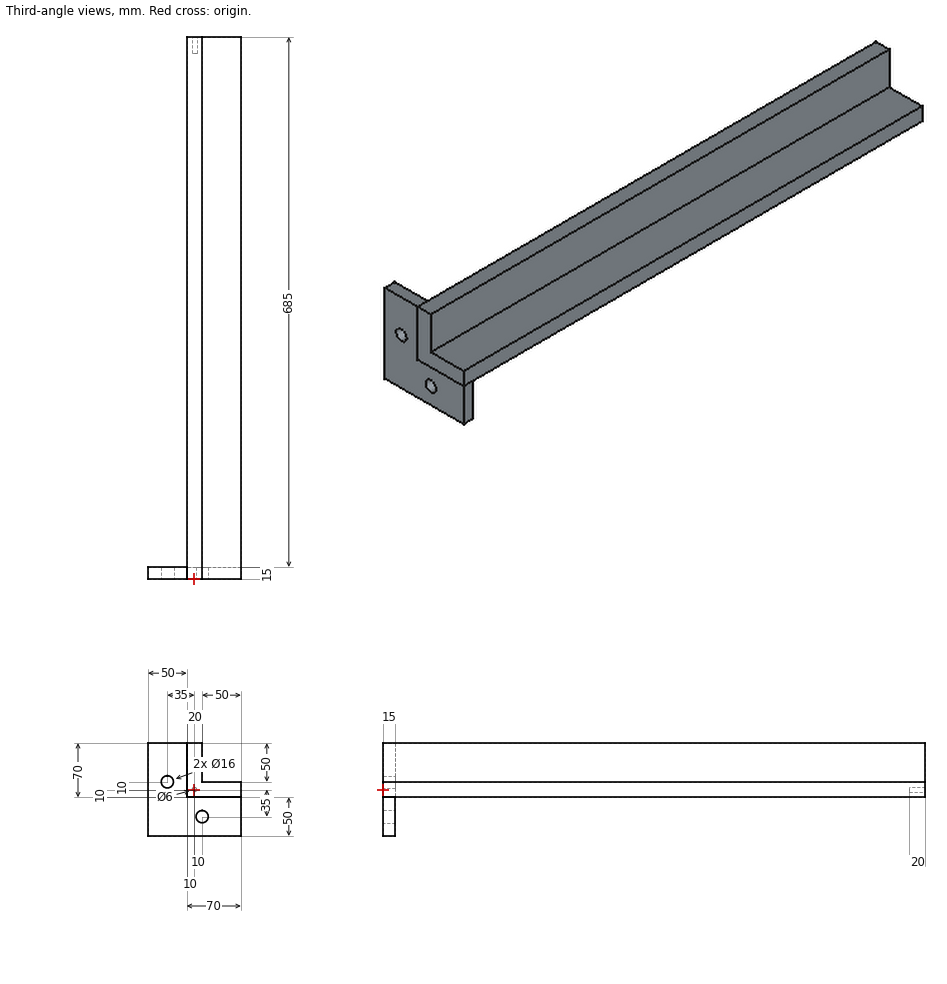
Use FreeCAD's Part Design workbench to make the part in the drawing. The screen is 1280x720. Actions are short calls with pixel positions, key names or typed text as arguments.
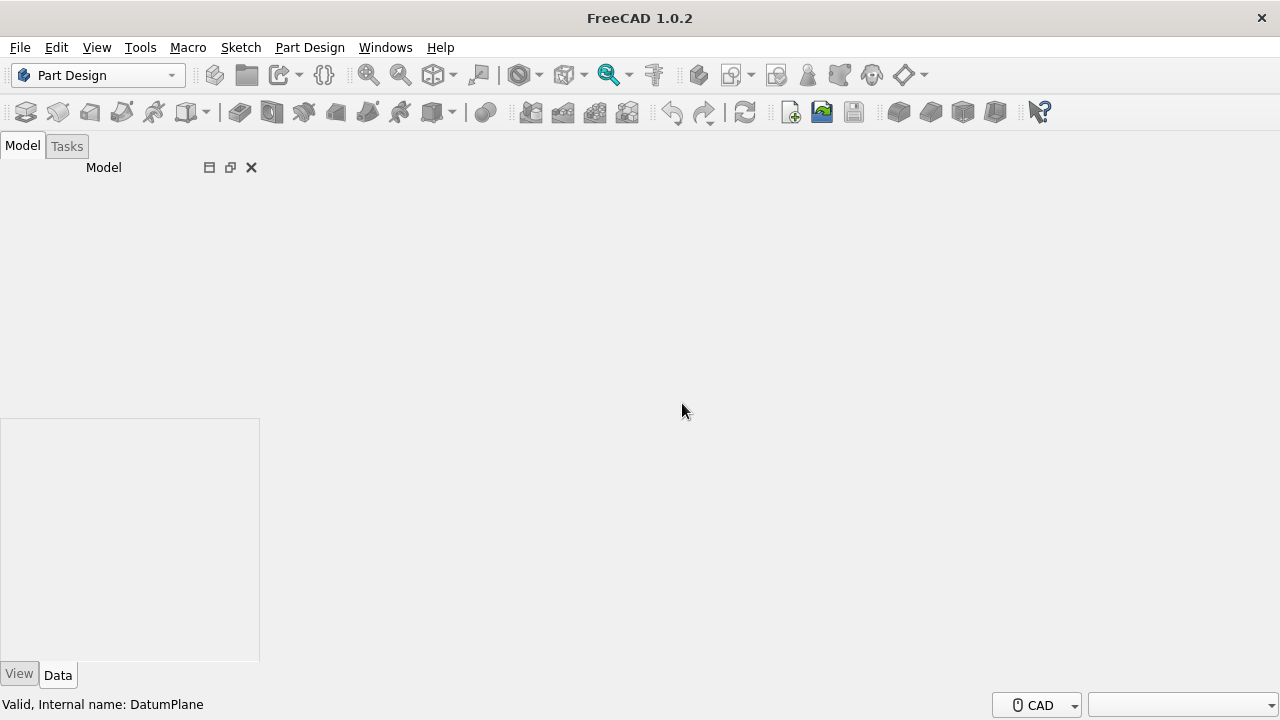
click(790, 112)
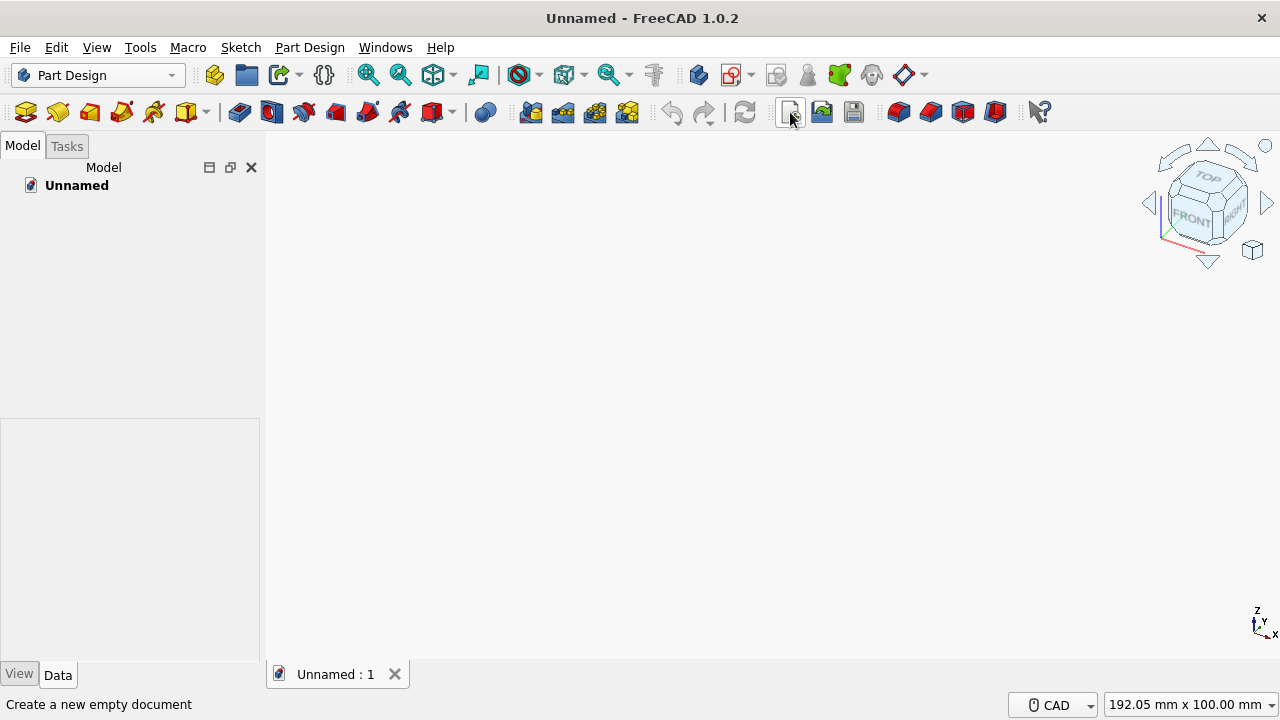
click(732, 76)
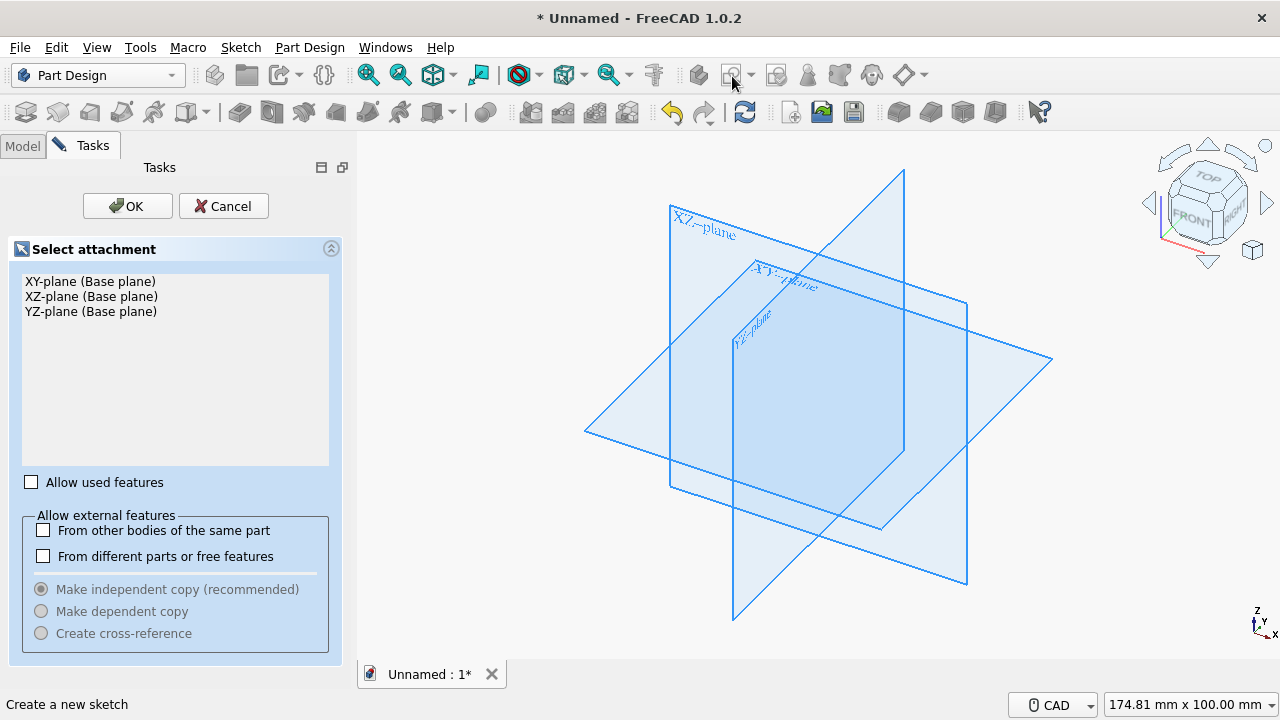
click(82, 296)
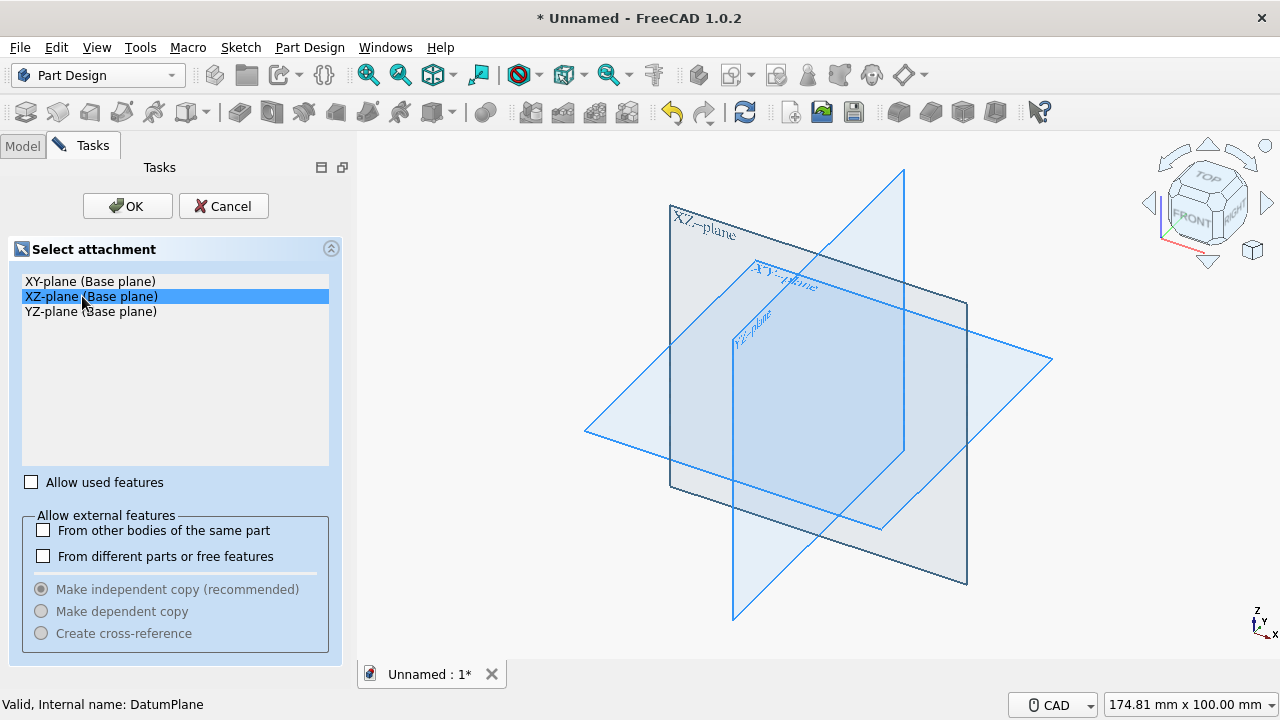
click(128, 206)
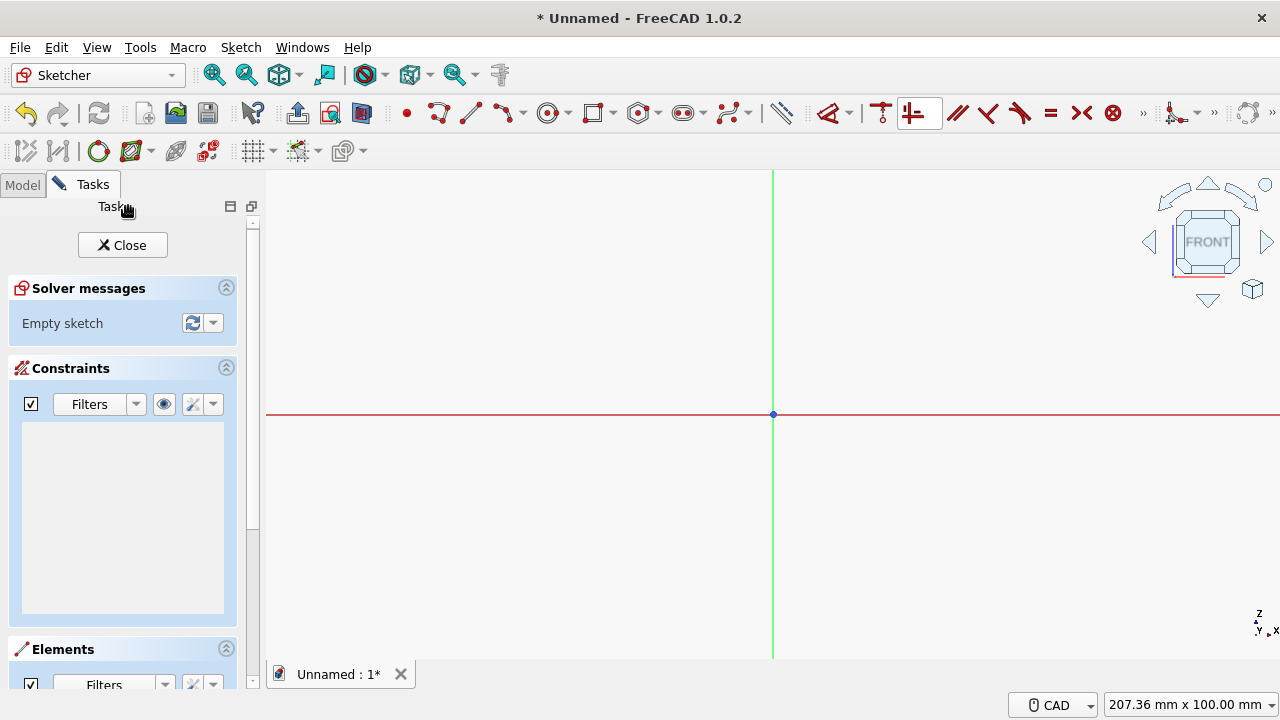
scroll(621, 414, down, 3)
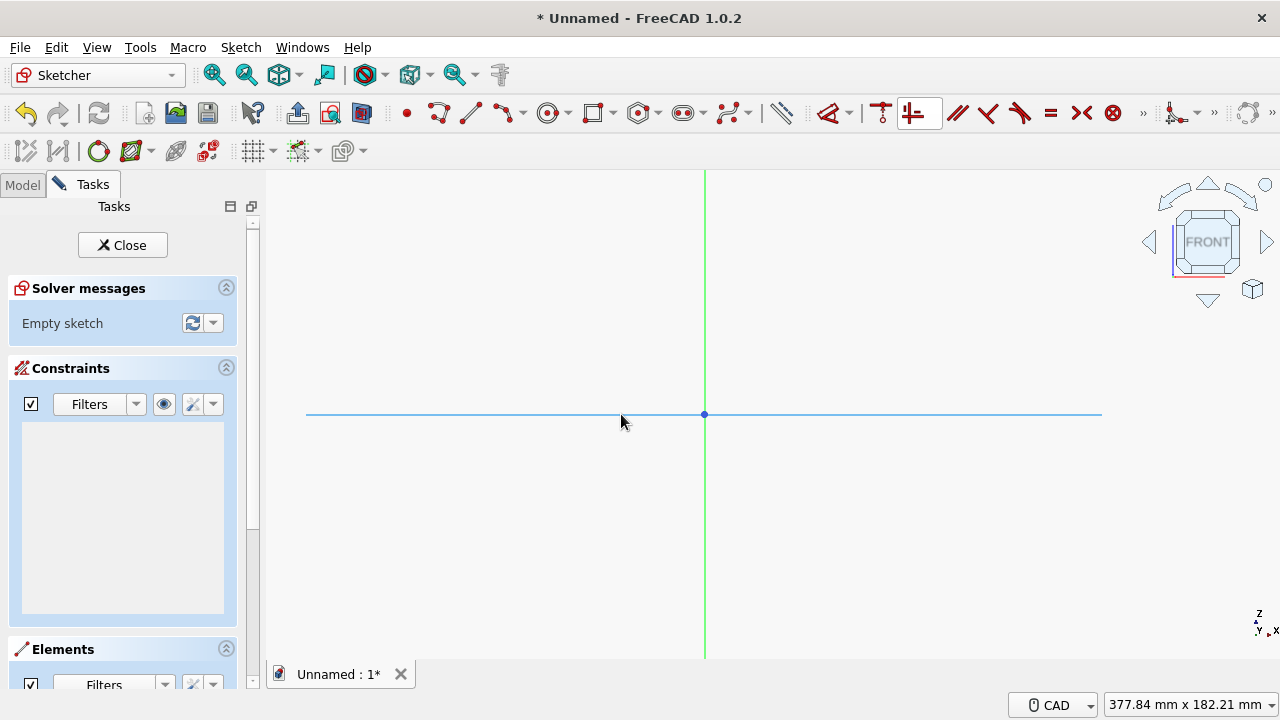
click(440, 114)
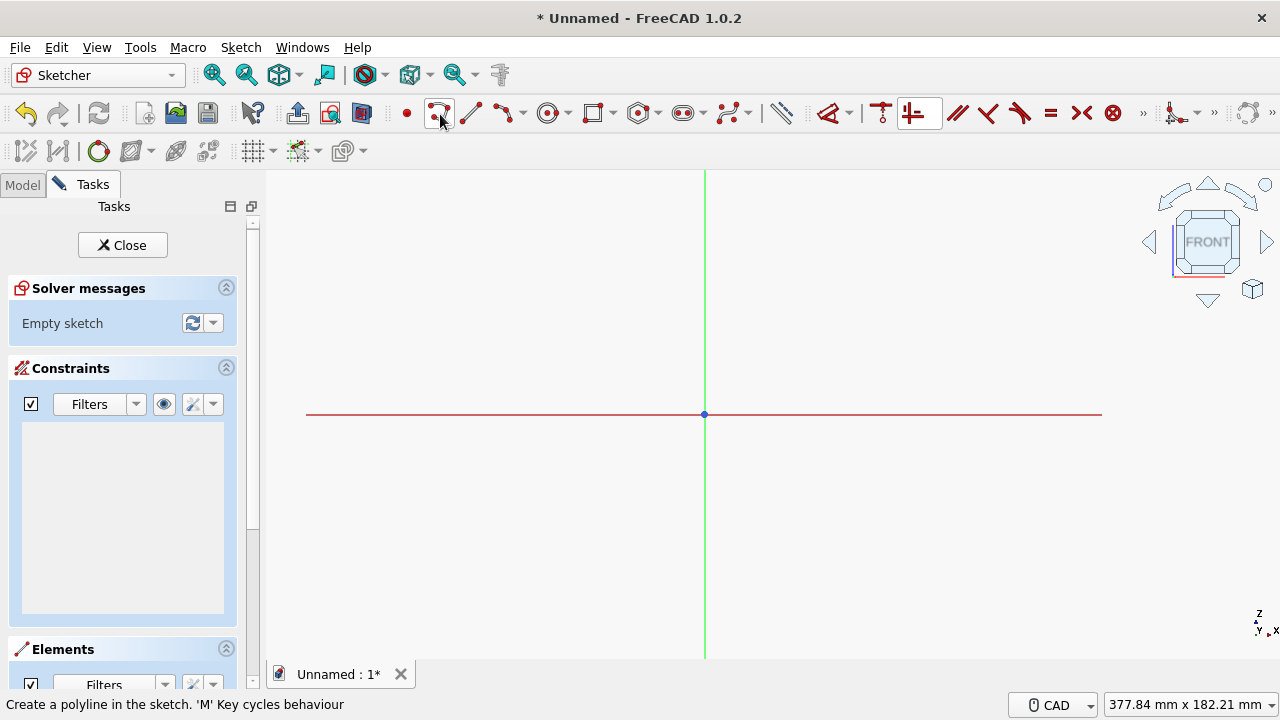
click(678, 441)
click(866, 441)
click(866, 576)
click(544, 576)
click(544, 253)
click(678, 253)
click(678, 442)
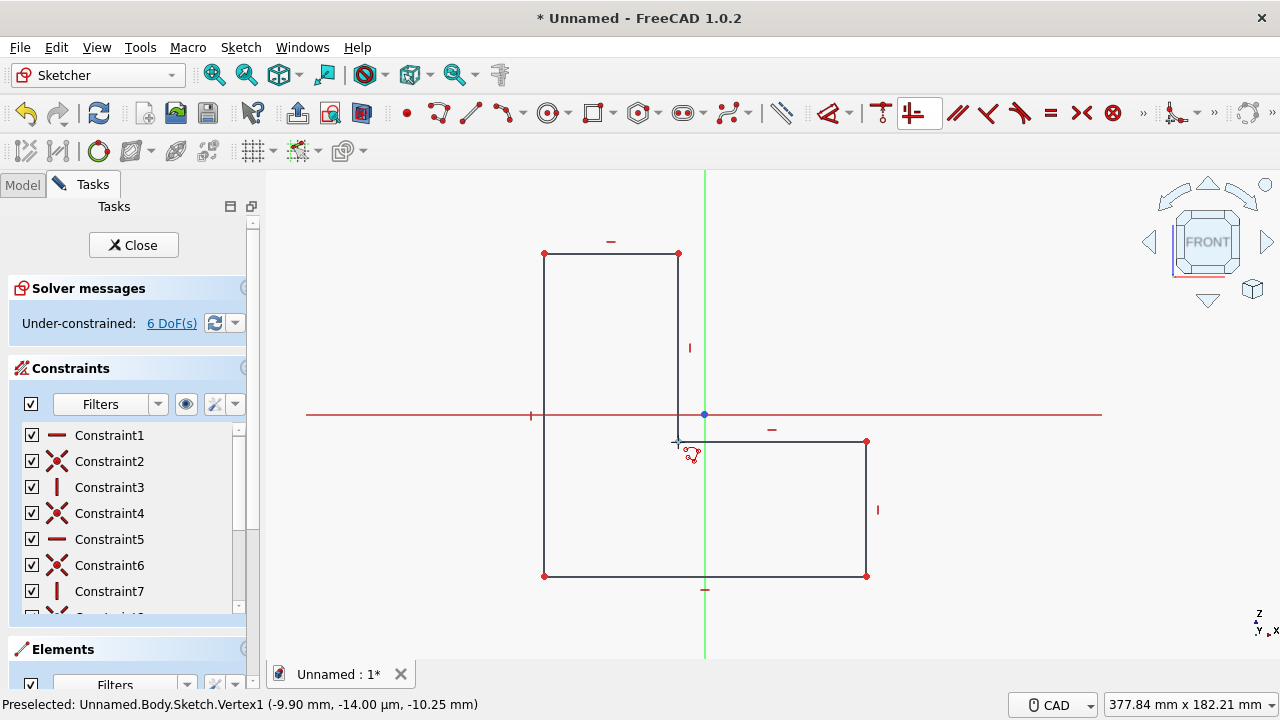
click(548, 114)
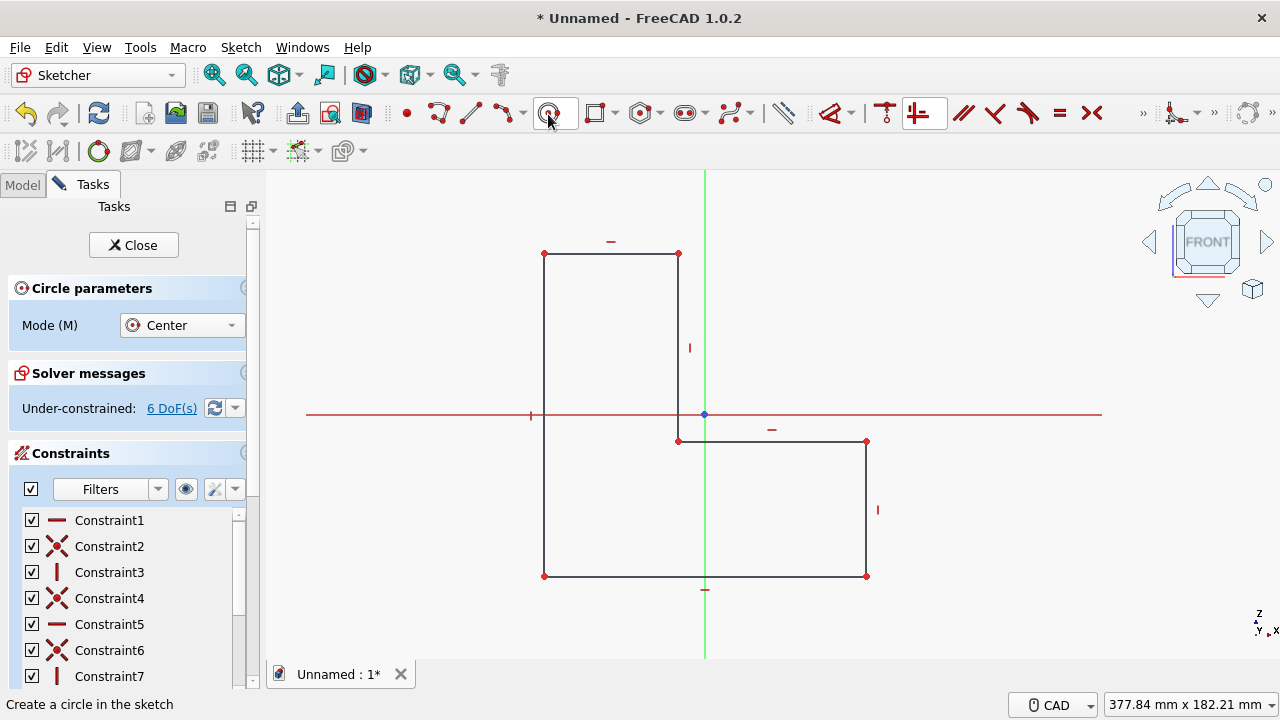
click(611, 388)
move(626, 372)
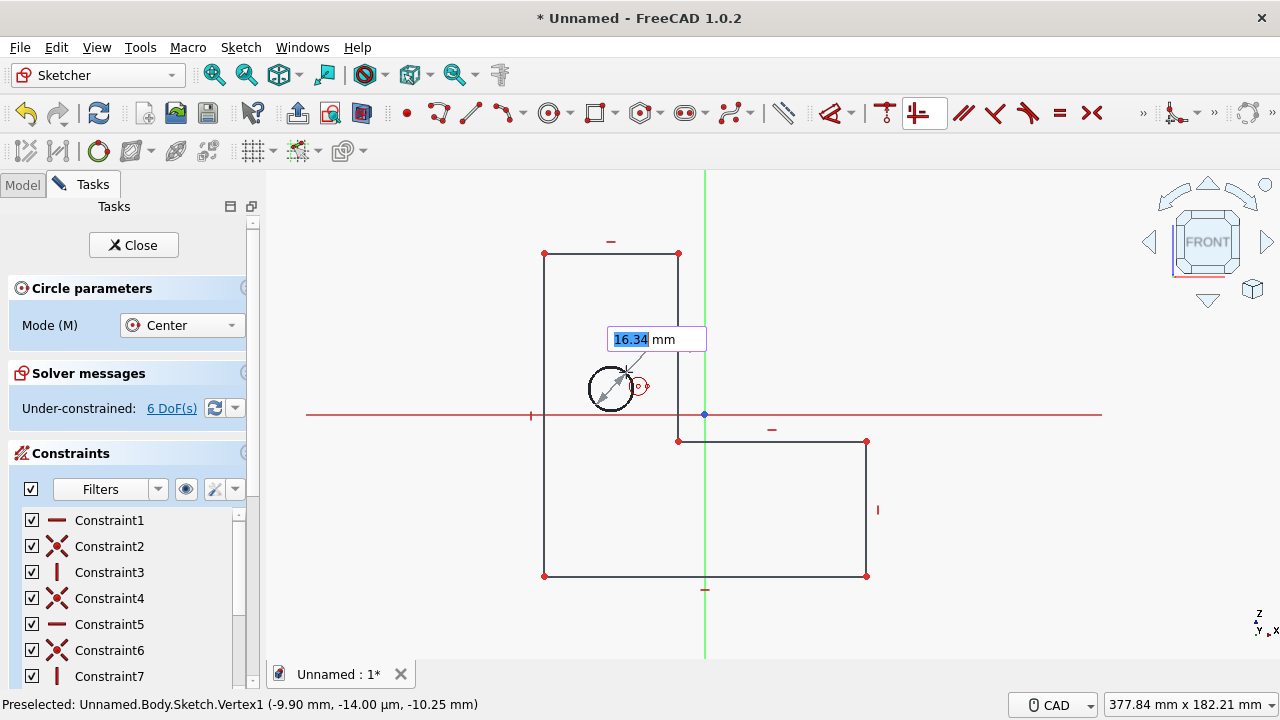
text(16)
key(Return)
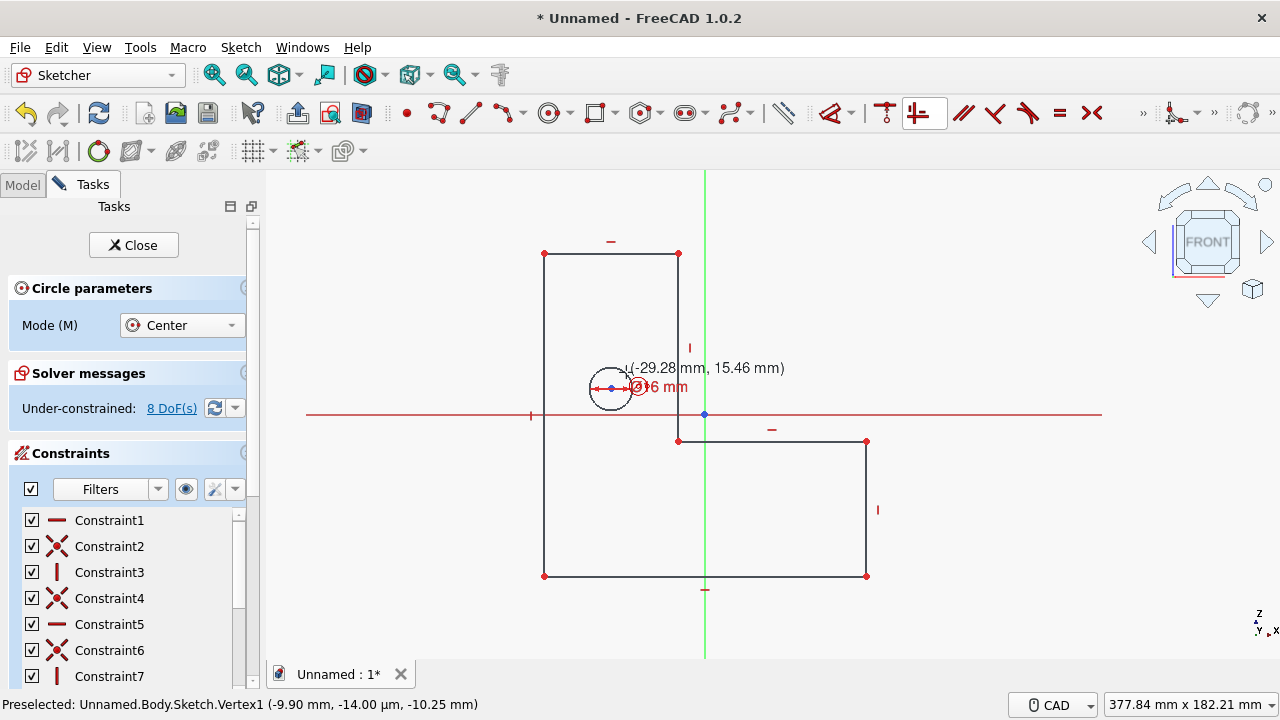
click(731, 508)
move(747, 493)